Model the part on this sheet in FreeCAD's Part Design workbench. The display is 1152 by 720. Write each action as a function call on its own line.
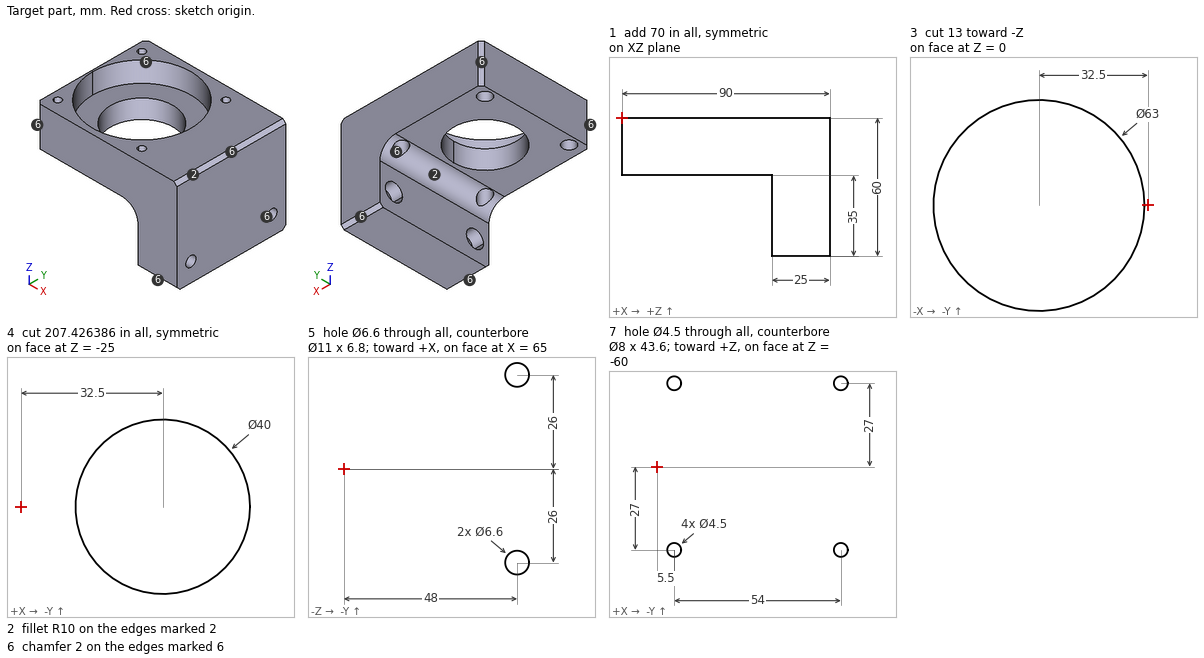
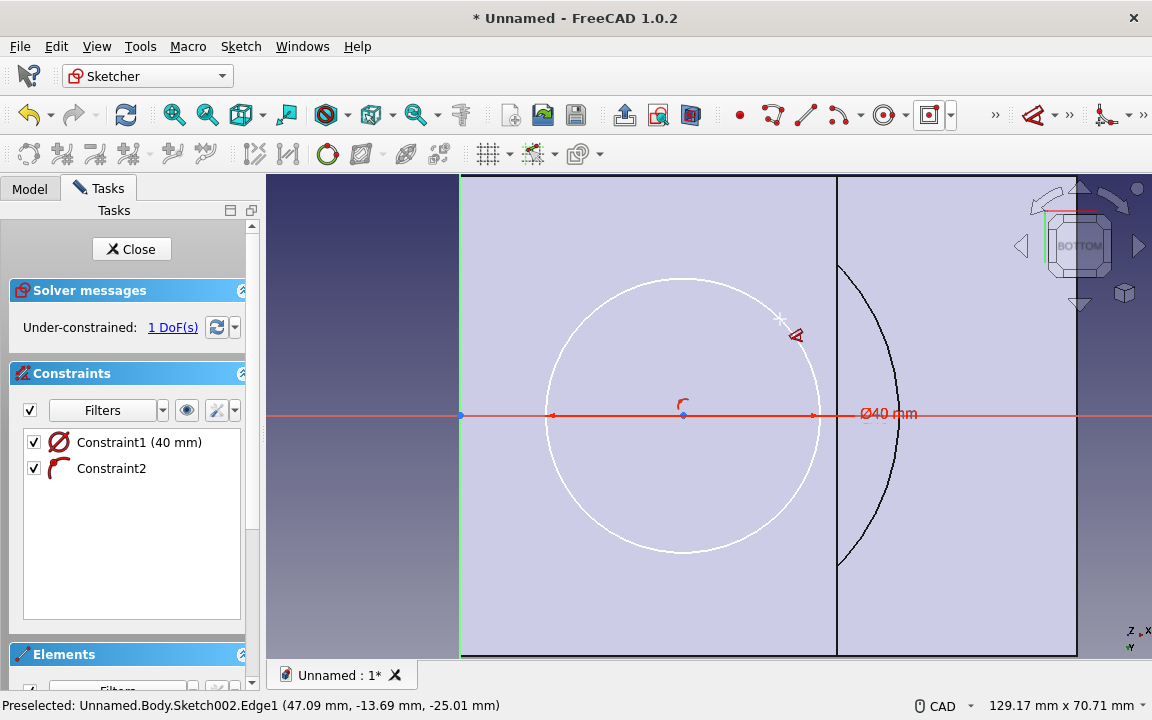
click(683, 416)
click(572, 450)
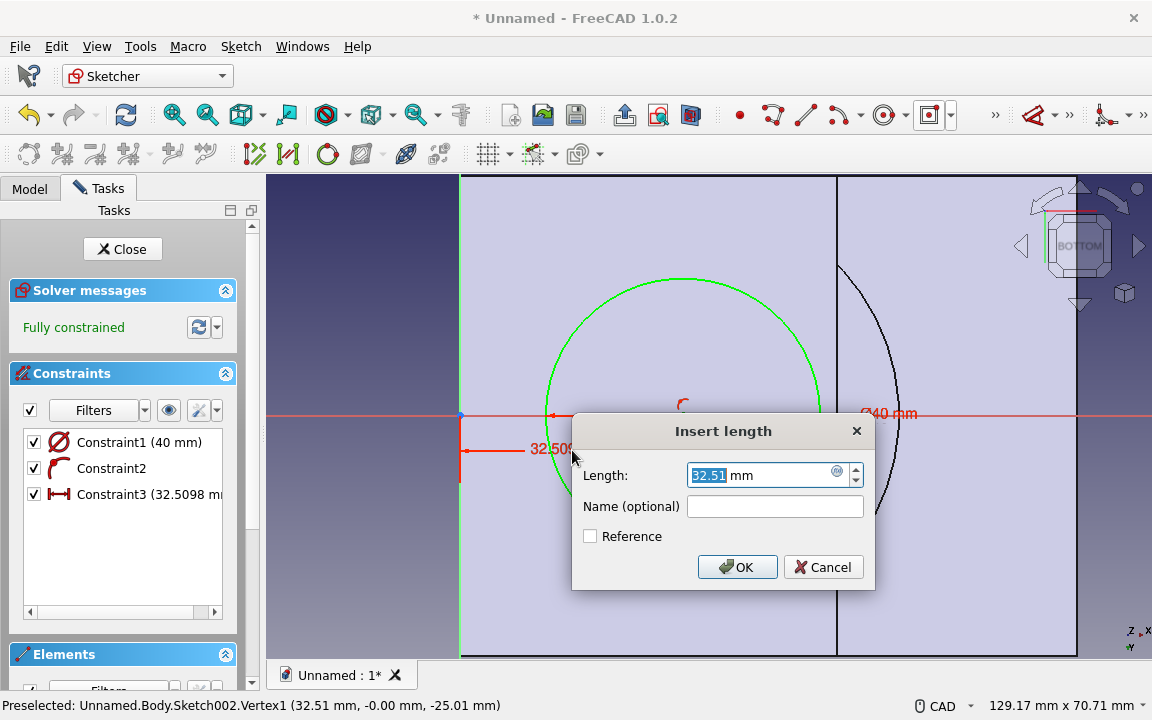
text(32.5)
key(Return)
key(Escape)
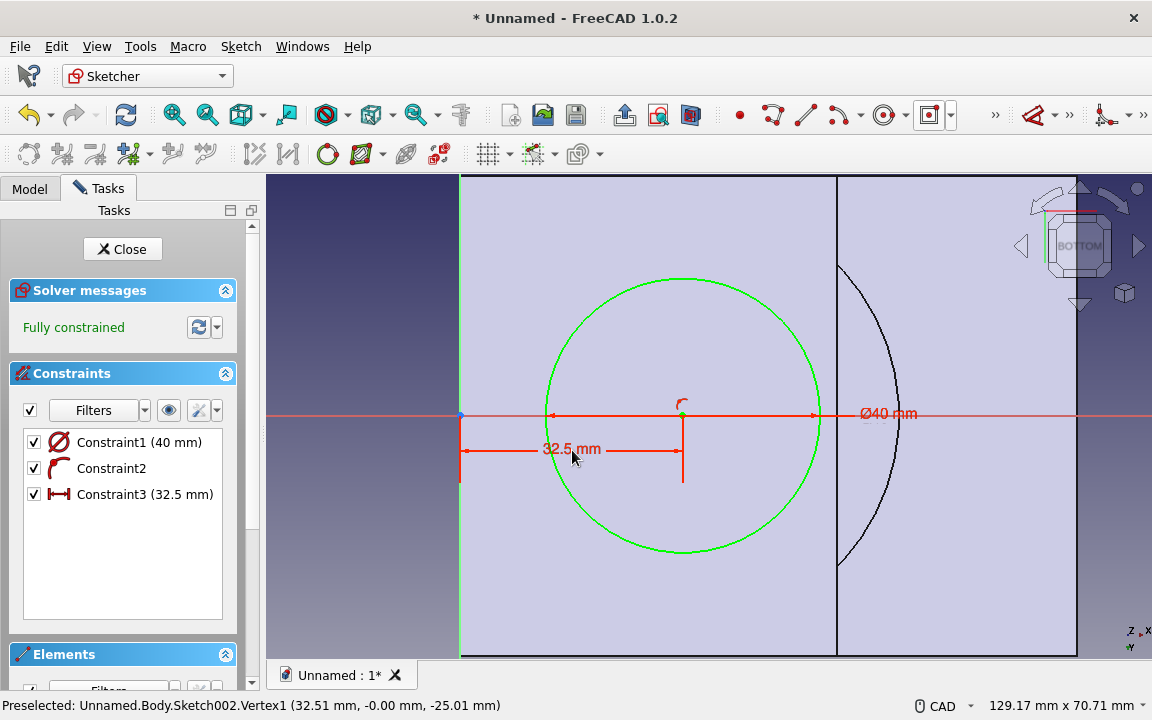
click(123, 249)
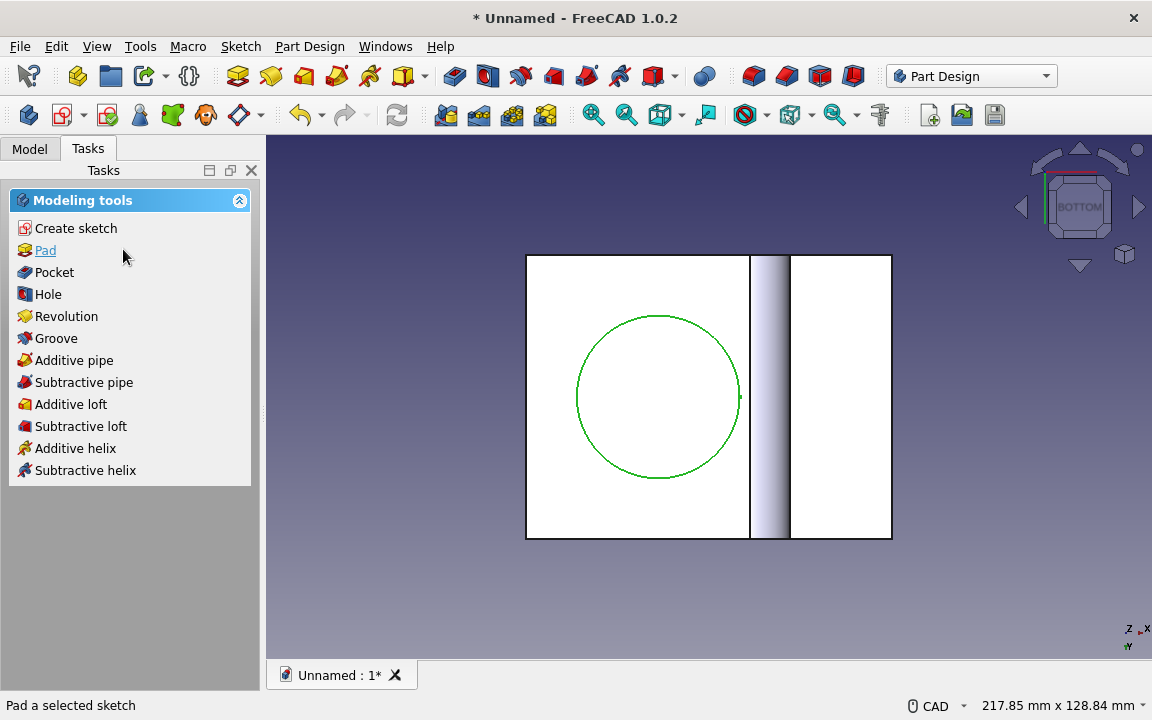
click(455, 76)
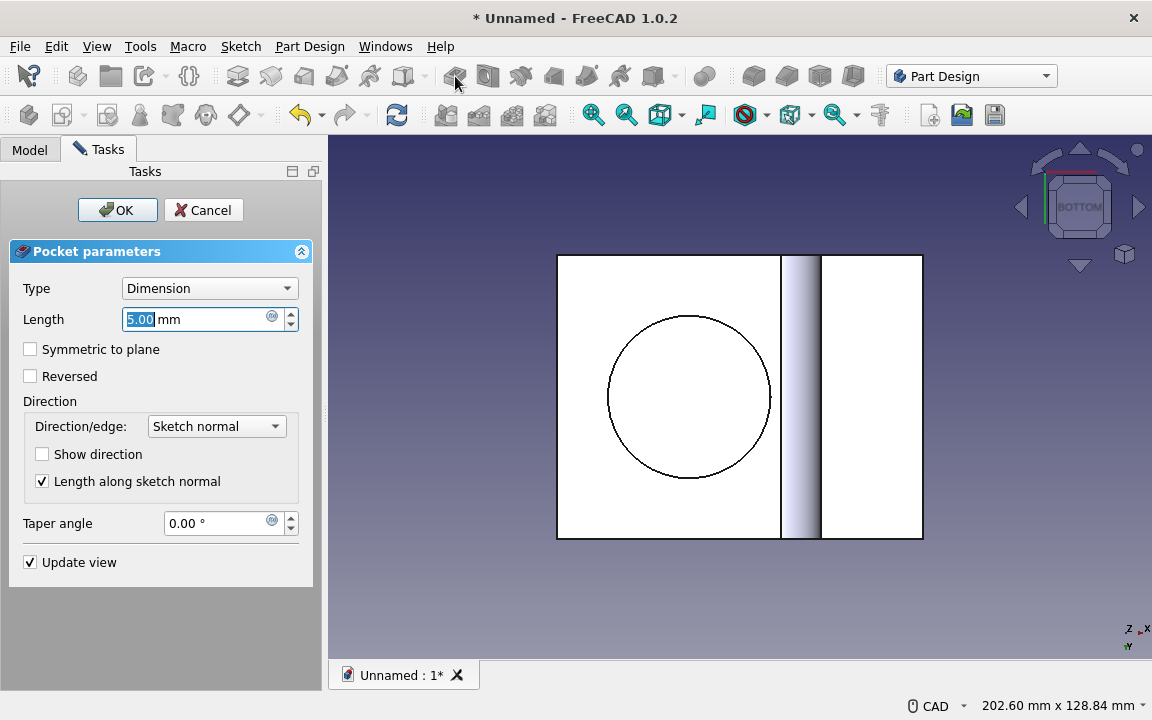
text(207.426386)
key(Tab)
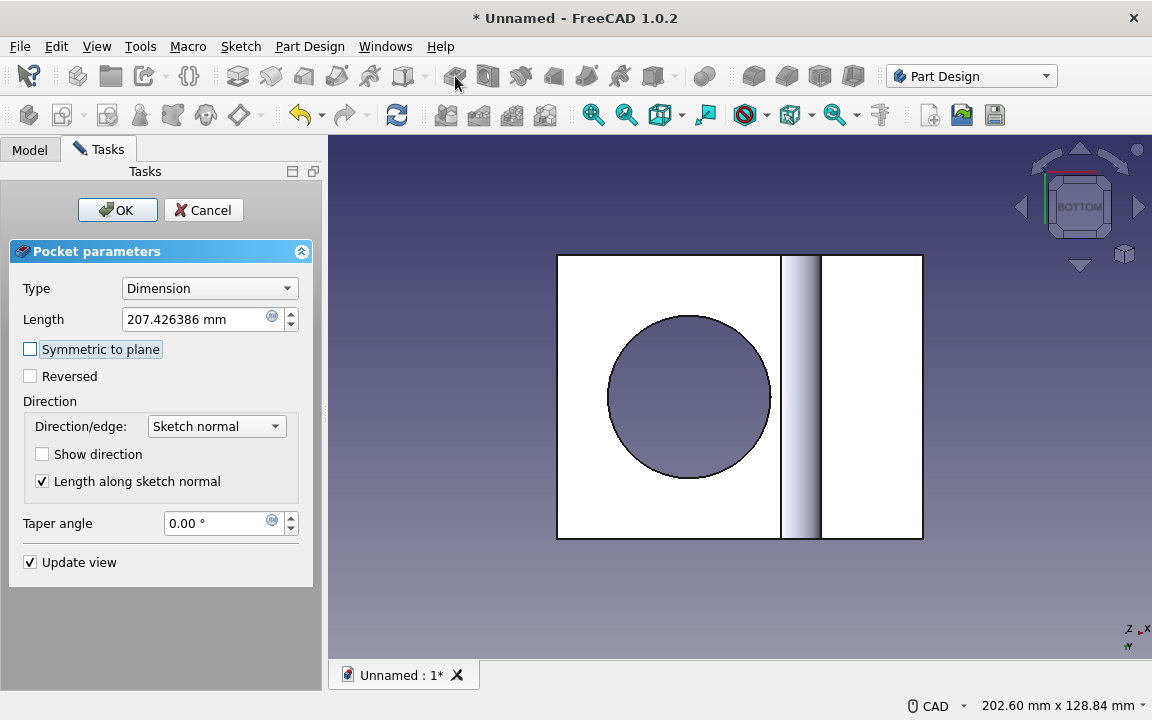
click(31, 349)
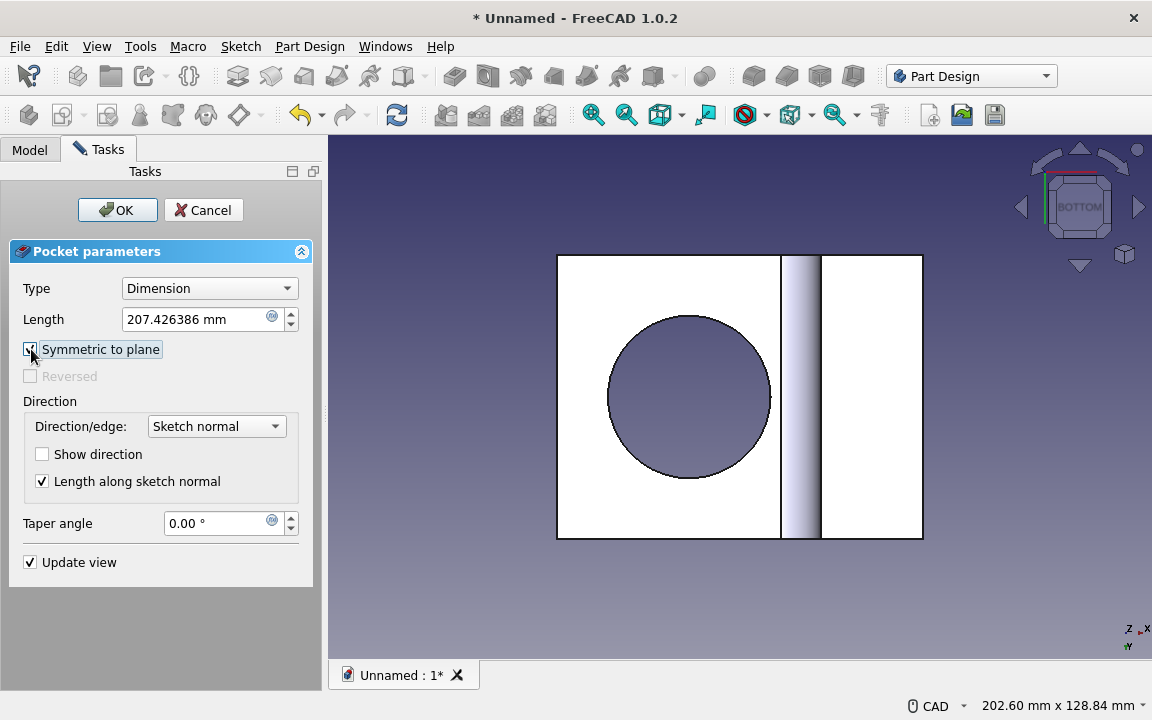
click(118, 210)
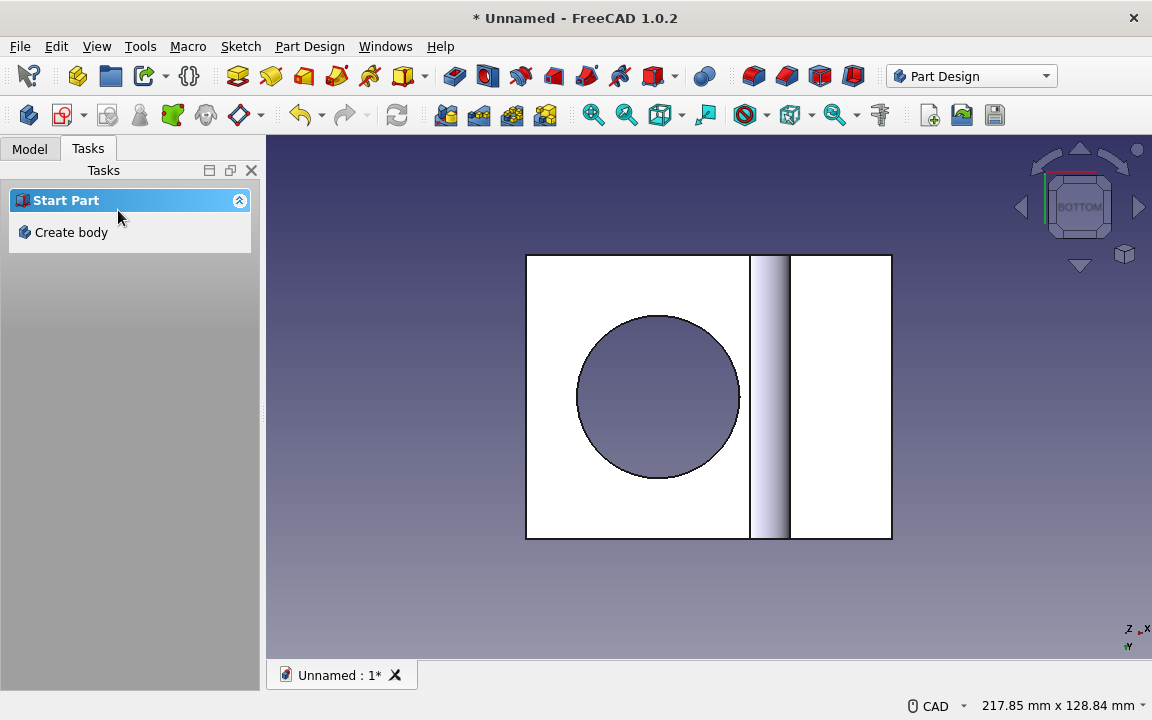
key(6)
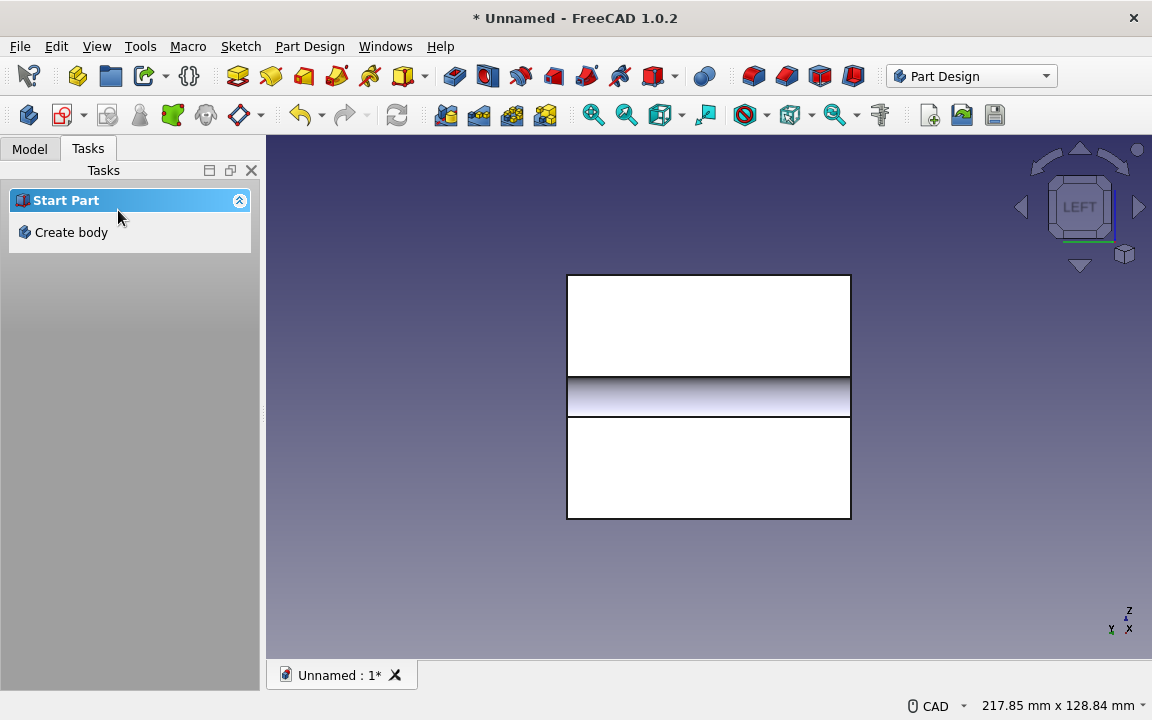
click(668, 467)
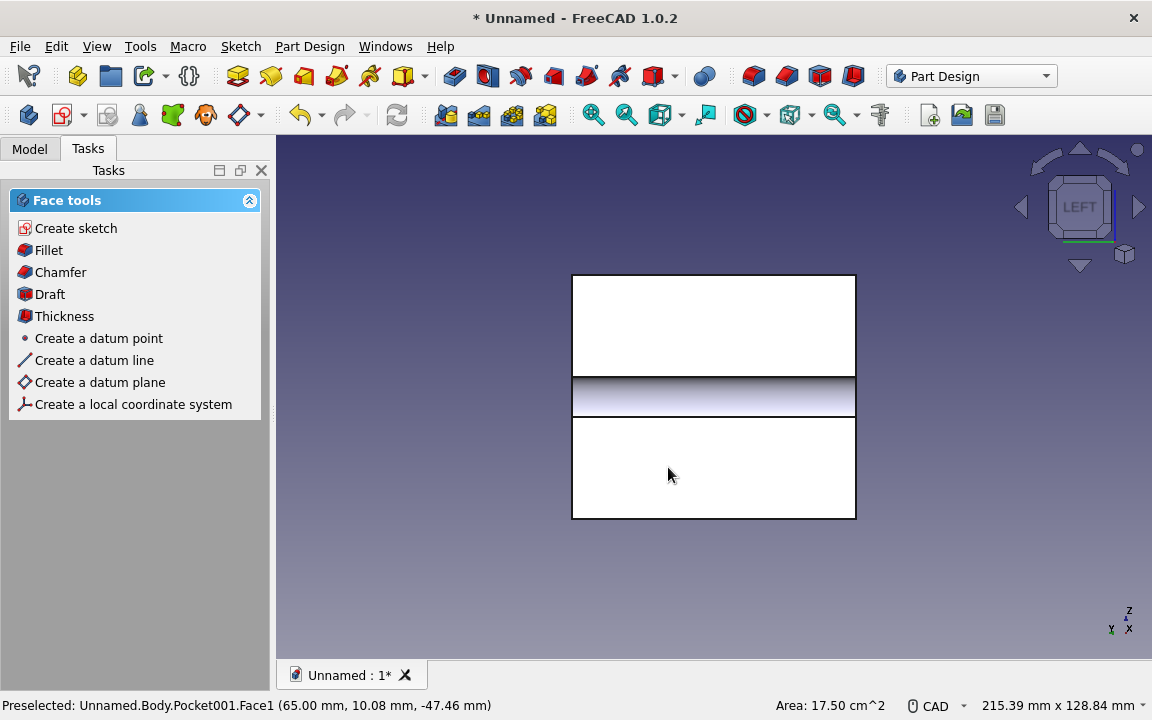
click(62, 116)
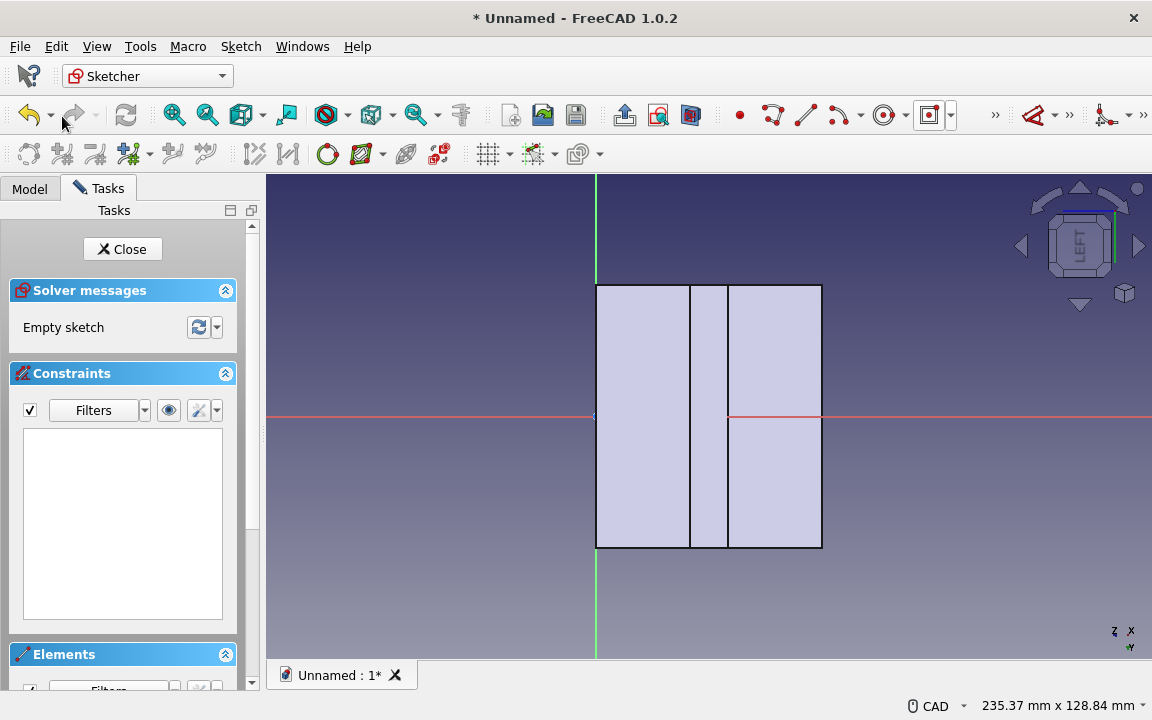
scroll(799, 417, up, 2)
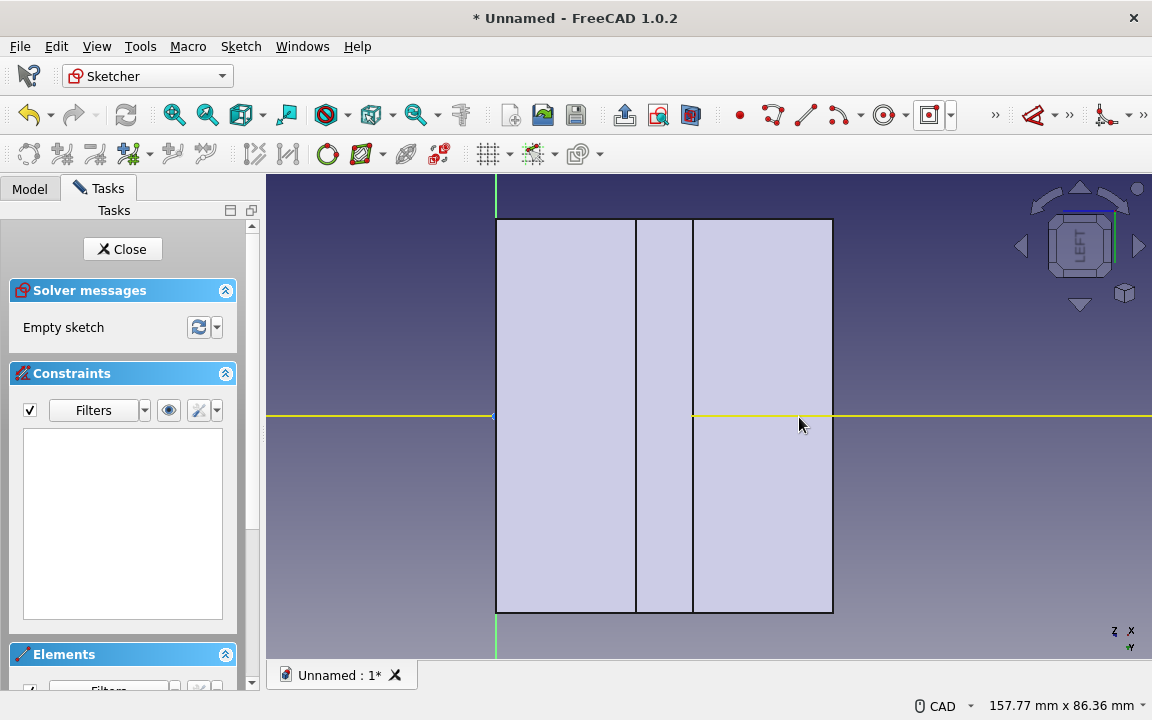
click(884, 116)